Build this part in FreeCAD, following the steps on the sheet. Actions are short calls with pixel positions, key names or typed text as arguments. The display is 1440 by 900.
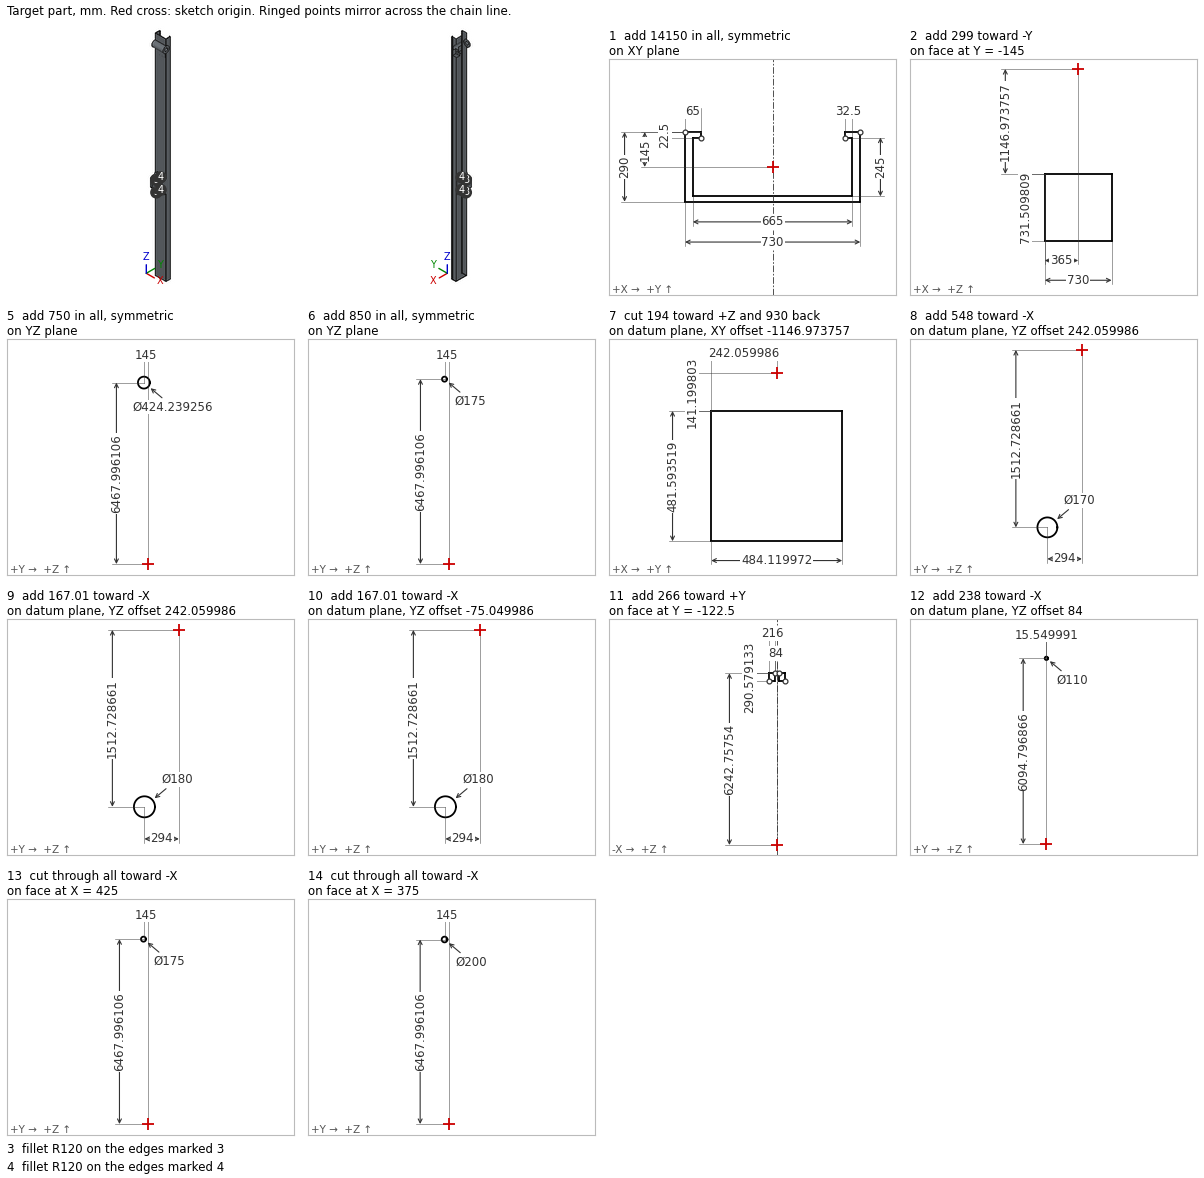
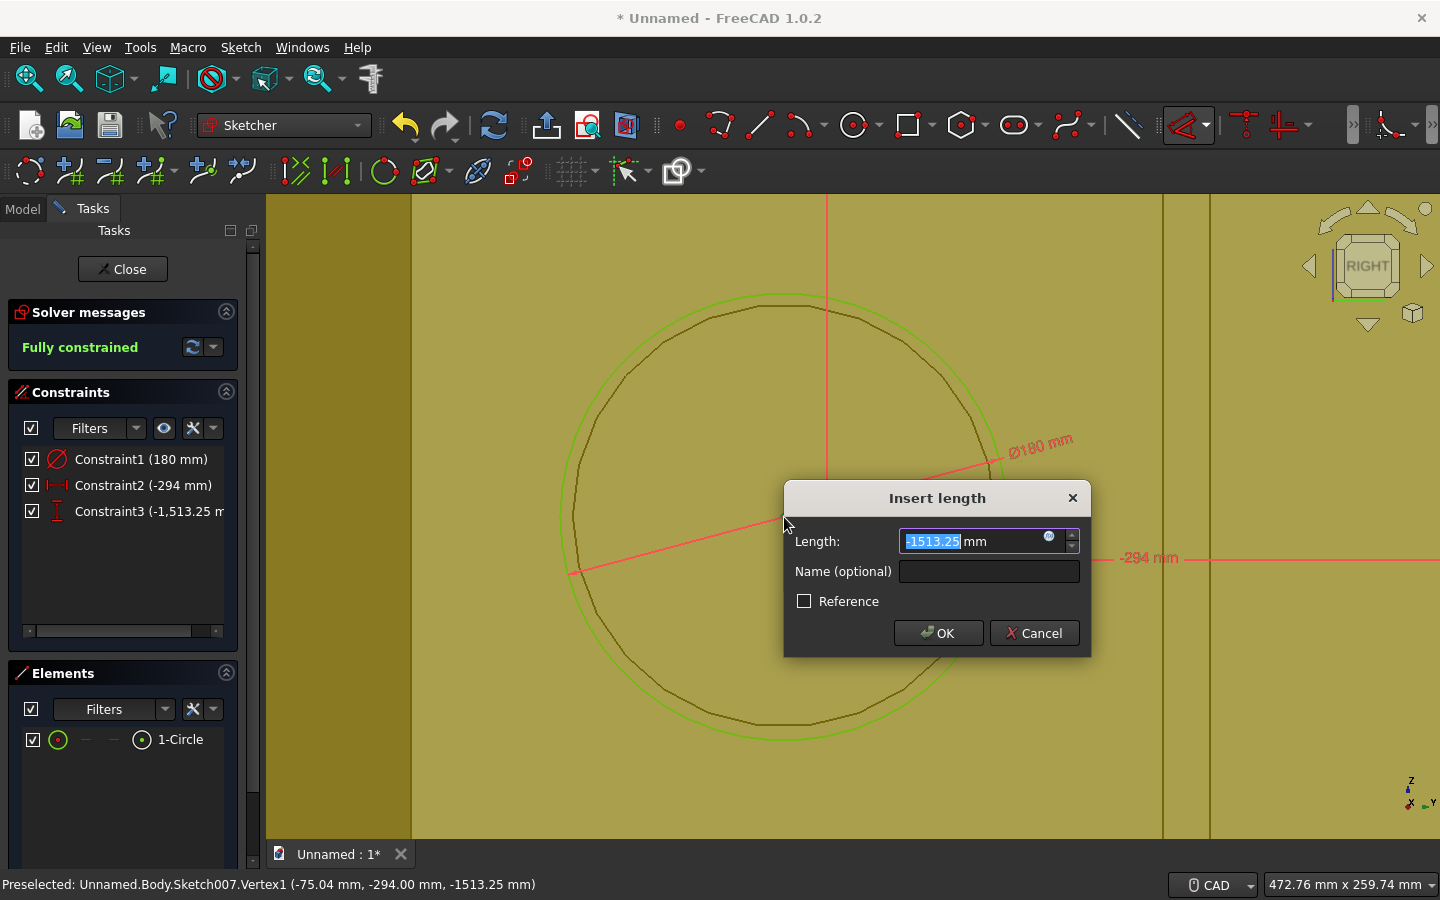
text(-1512.728661)
key(Return)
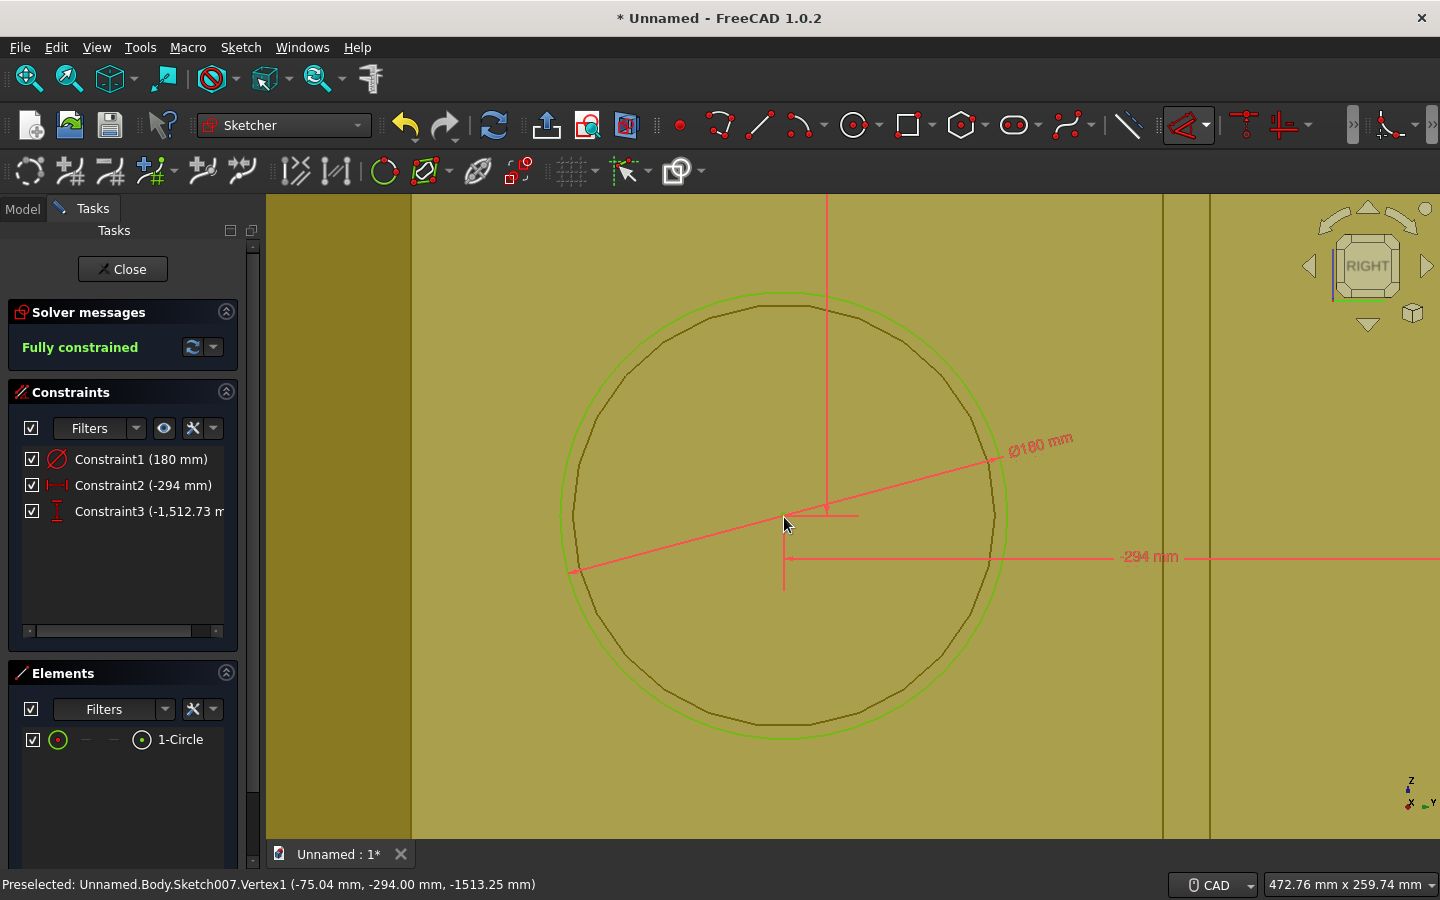
click(123, 269)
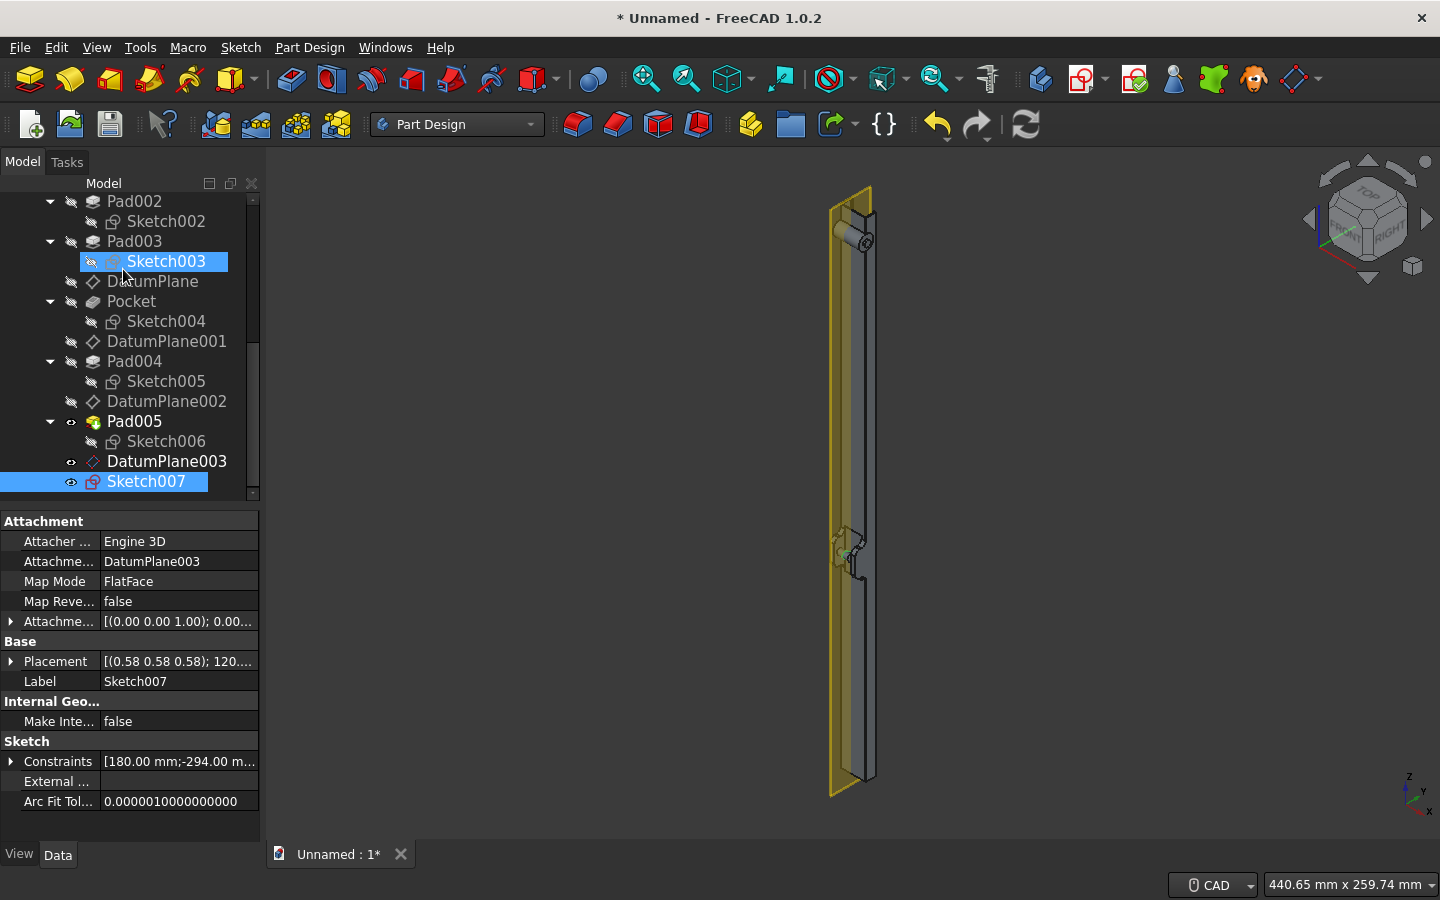
click(30, 80)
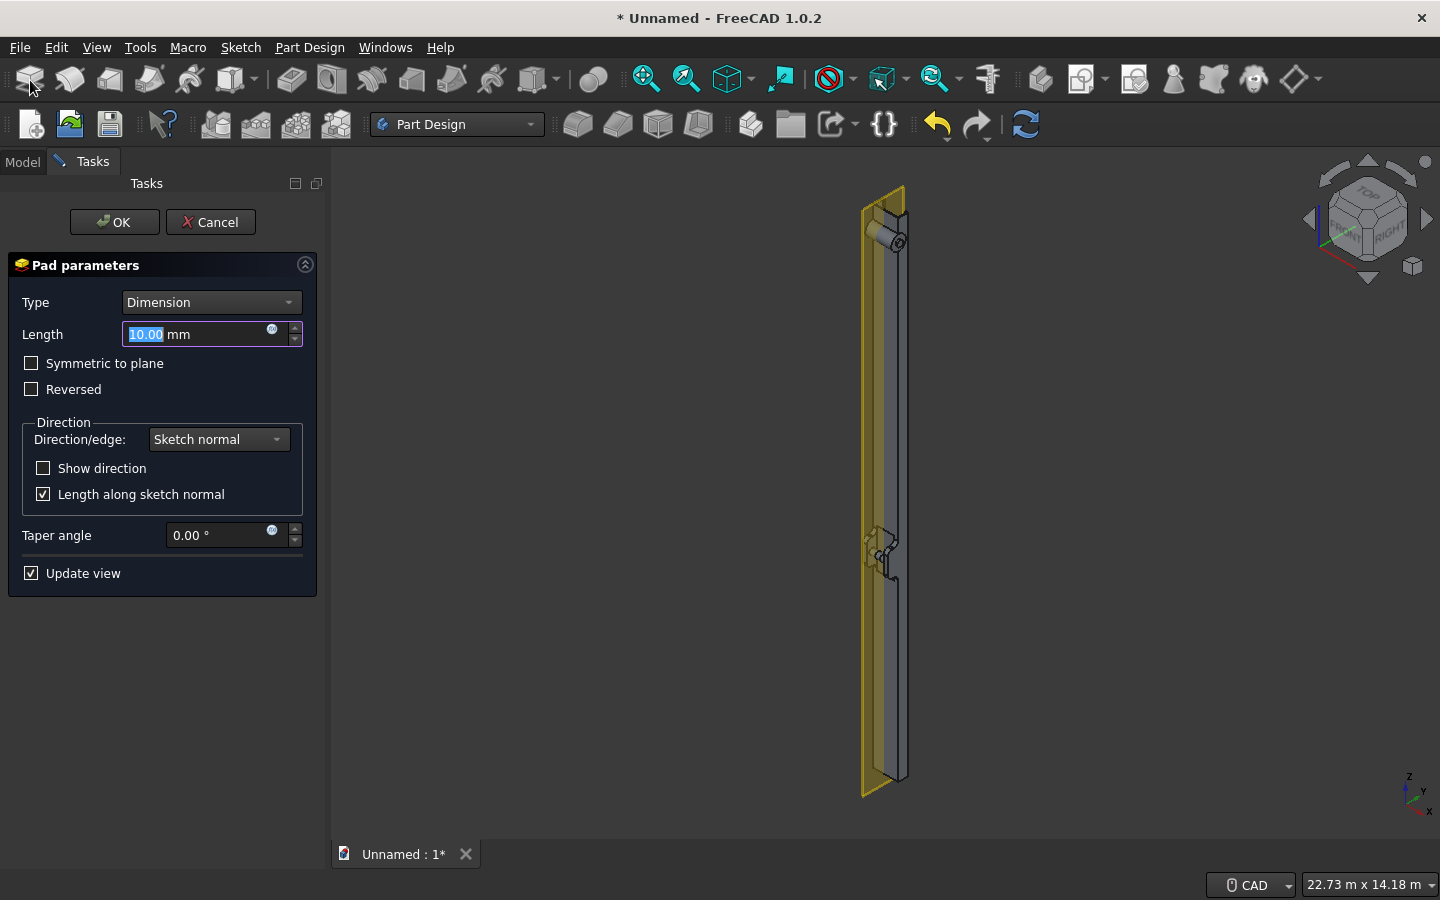
text(167.01)
key(Tab)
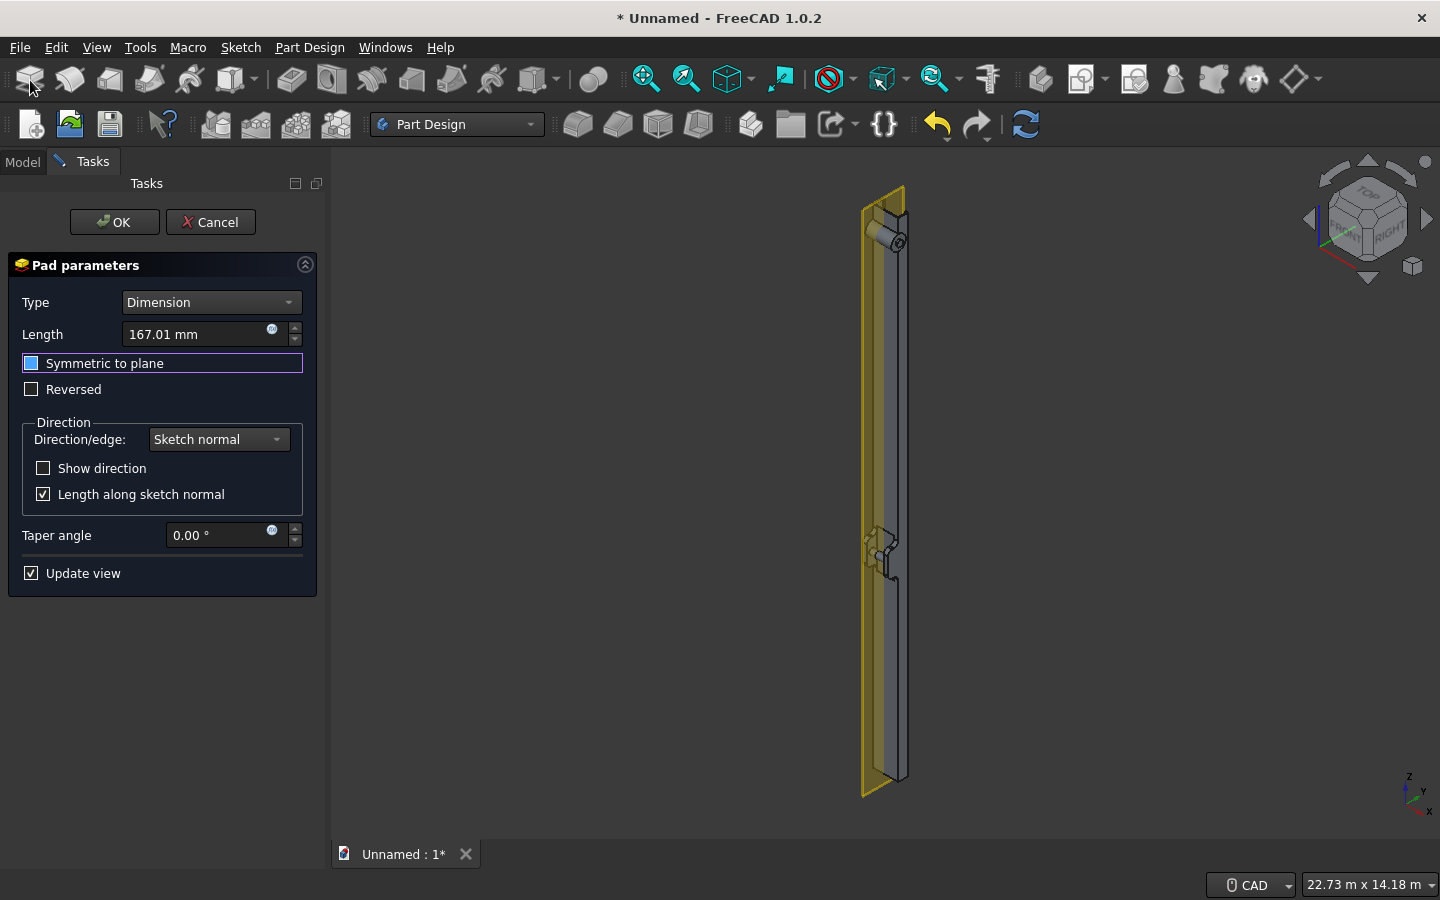
click(30, 389)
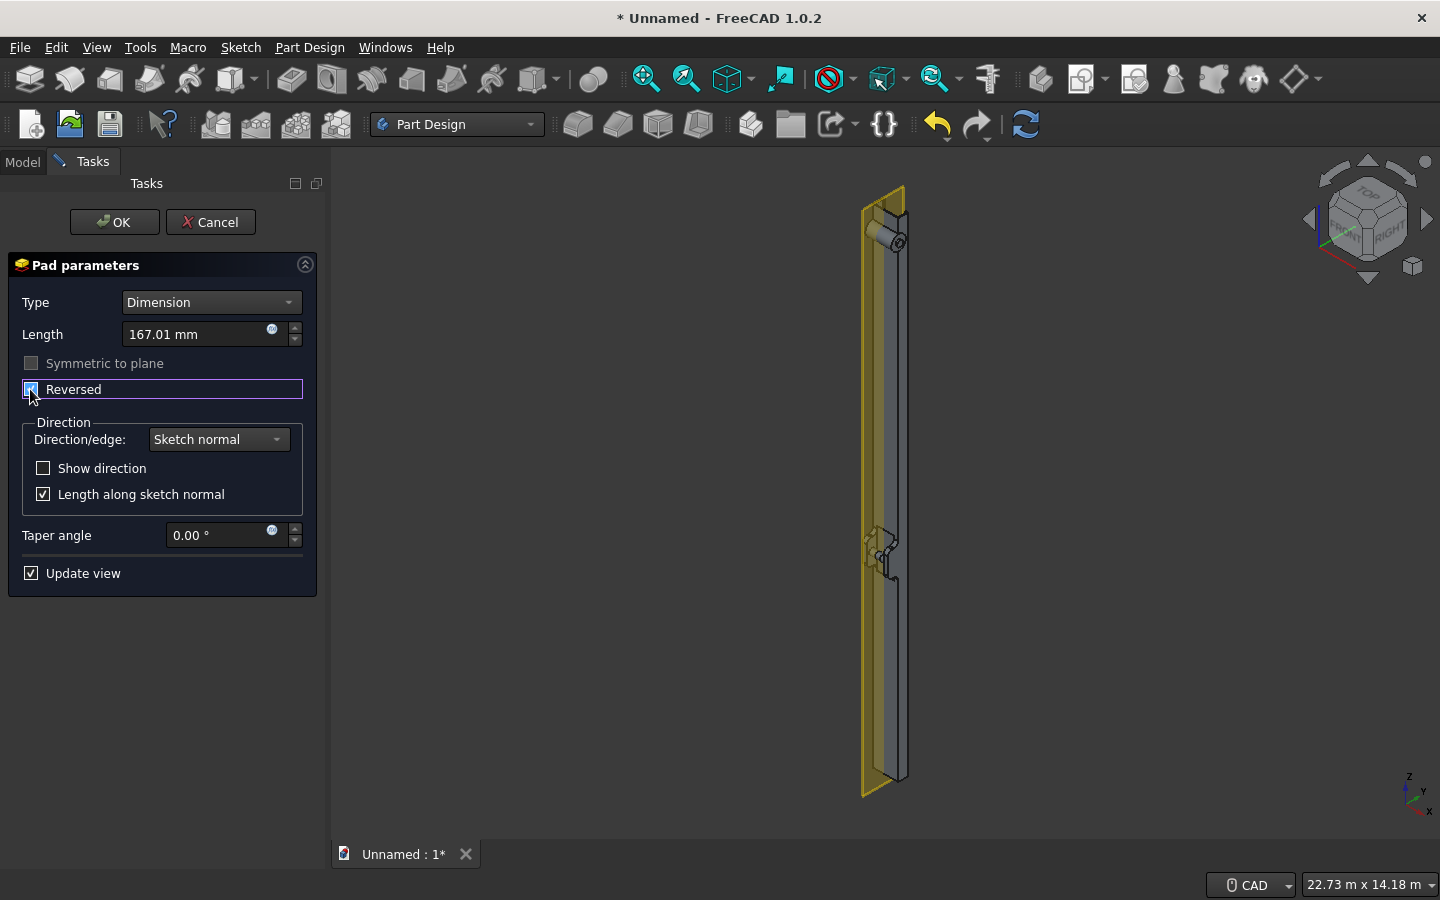
click(115, 222)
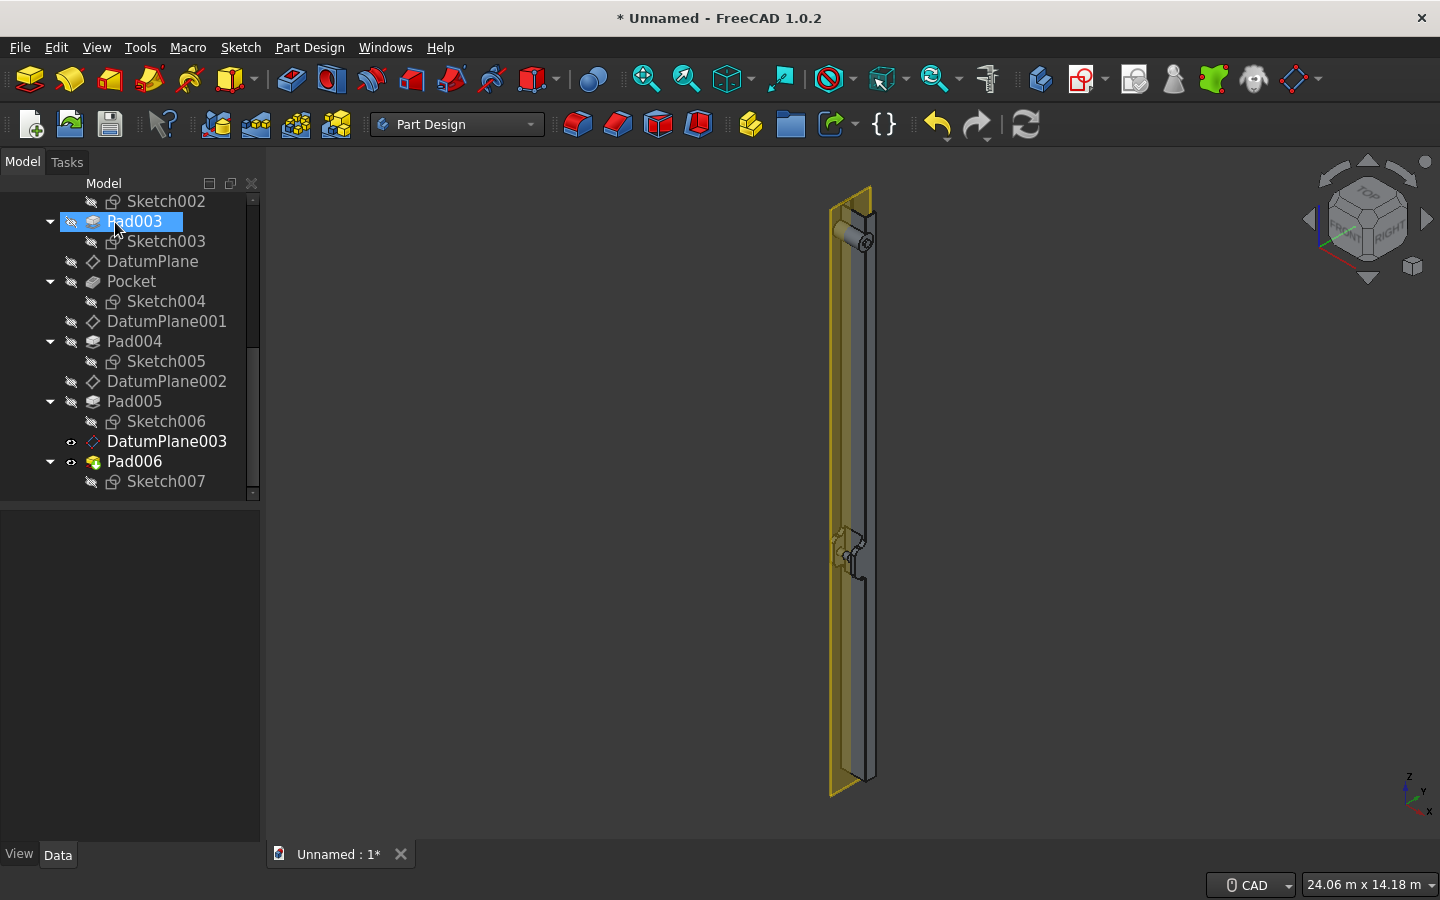
click(116, 442)
key(space)